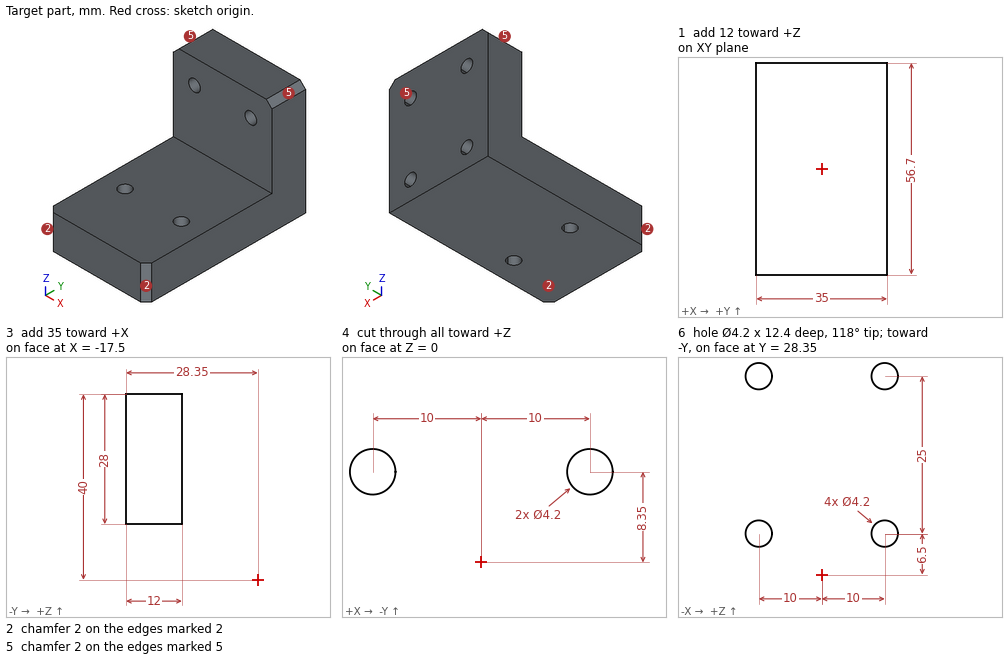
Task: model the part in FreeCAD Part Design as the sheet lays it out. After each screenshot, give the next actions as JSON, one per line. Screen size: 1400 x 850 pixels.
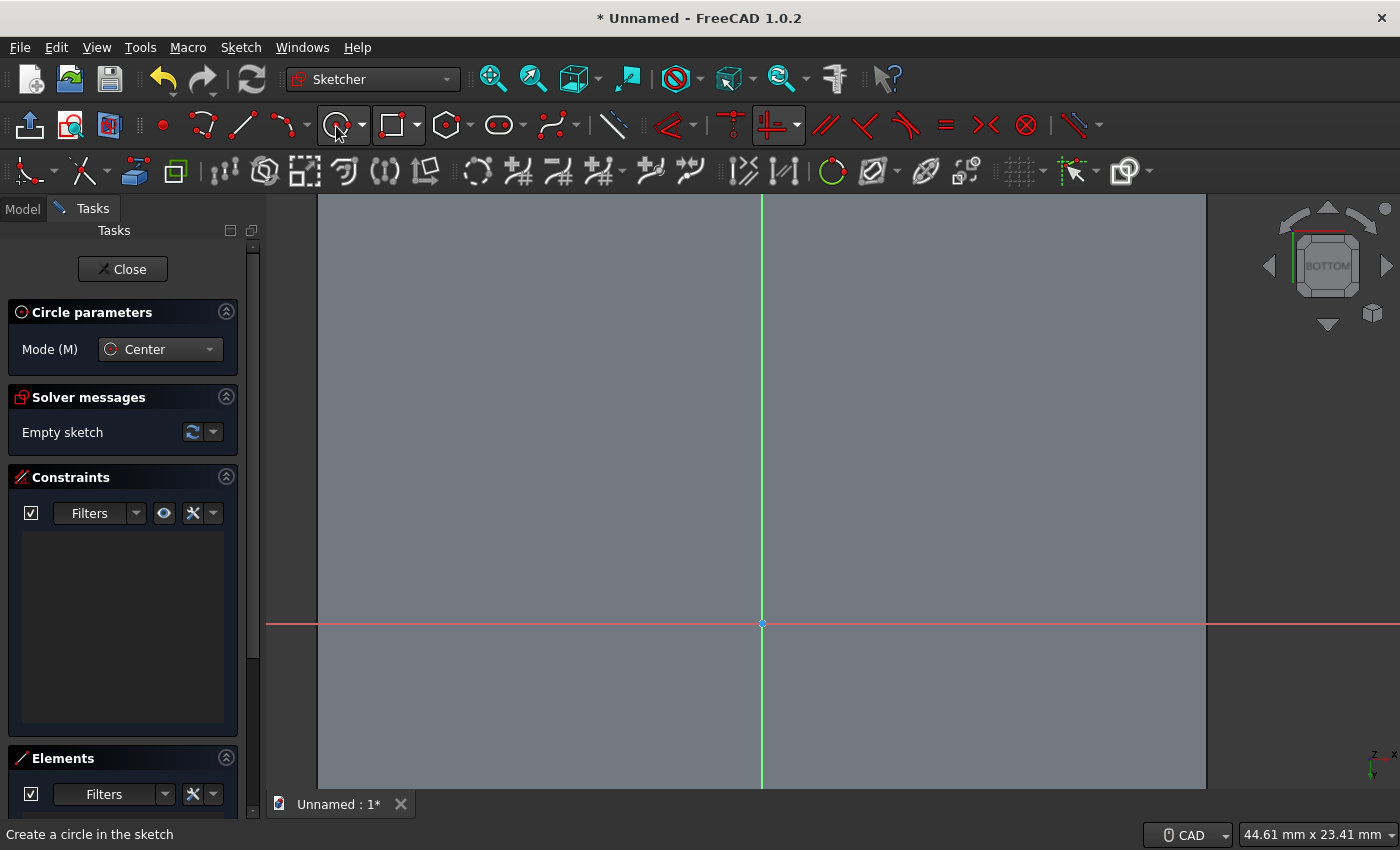
{"action": "left_click", "coordinate": [1016, 412]}
{"action": "left_click", "coordinate": [1054, 374]}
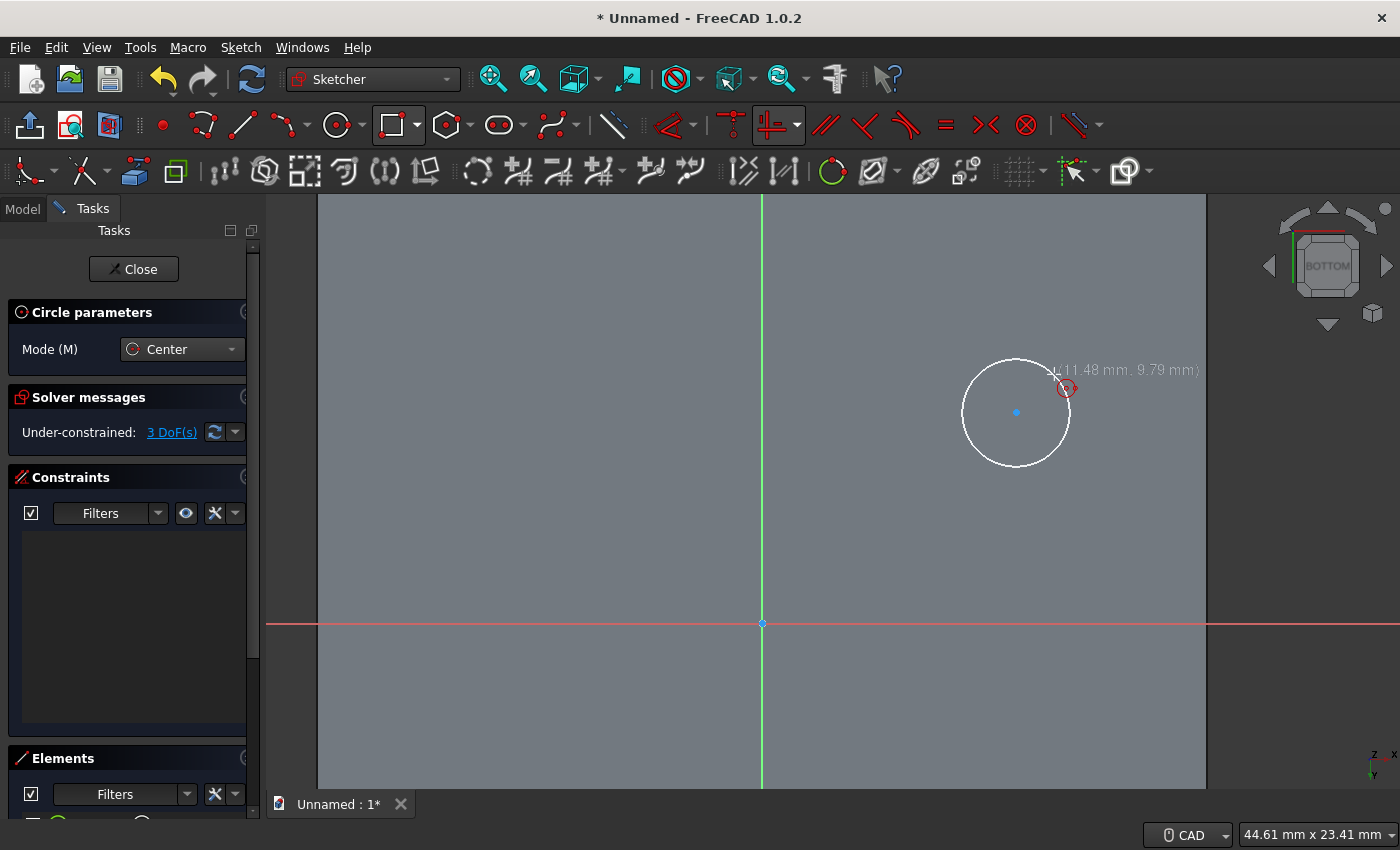
{"action": "left_click", "coordinate": [508, 412]}
{"action": "left_click", "coordinate": [546, 374]}
{"action": "key", "text": "Escape"}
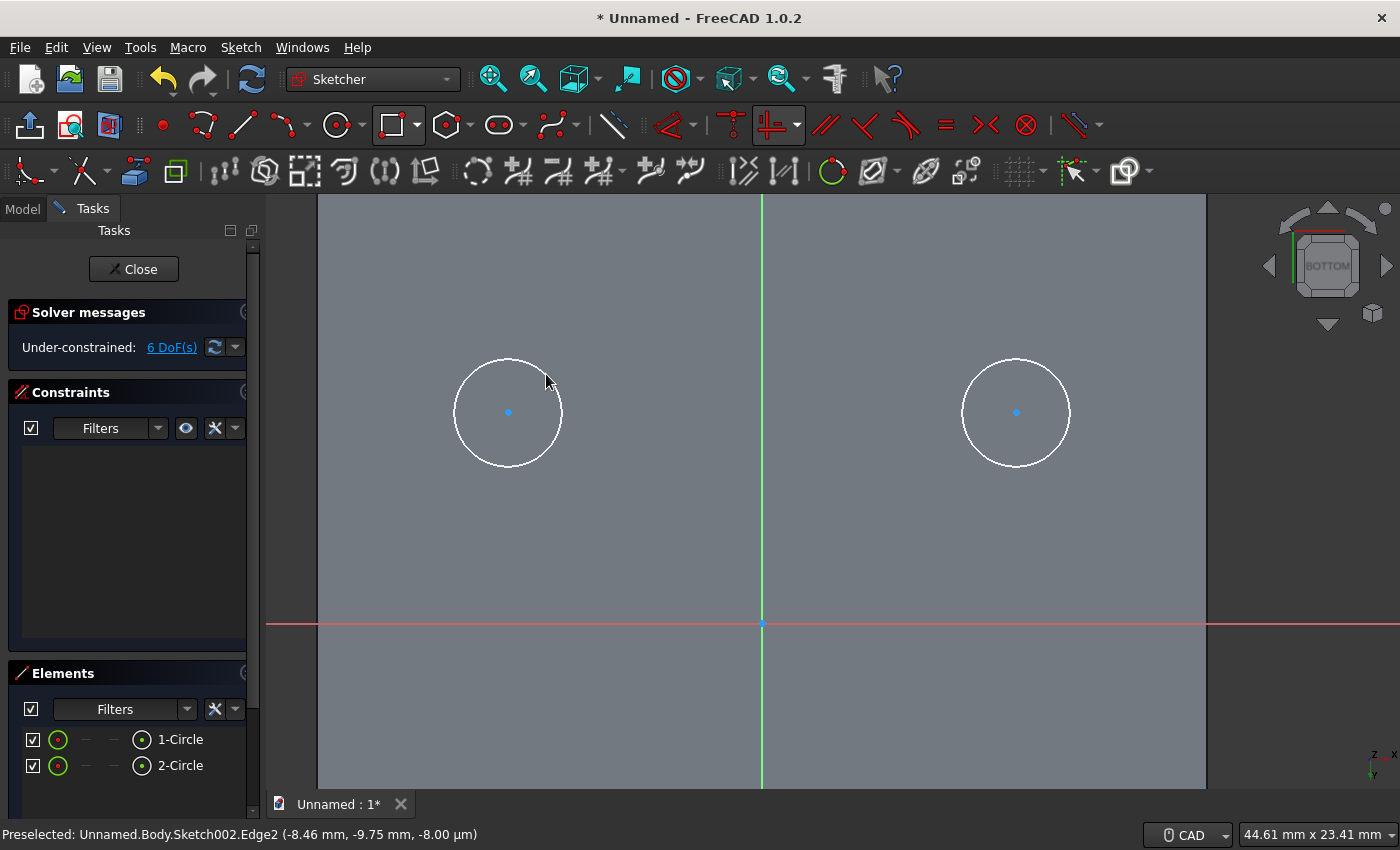
{"action": "left_click", "coordinate": [1054, 375]}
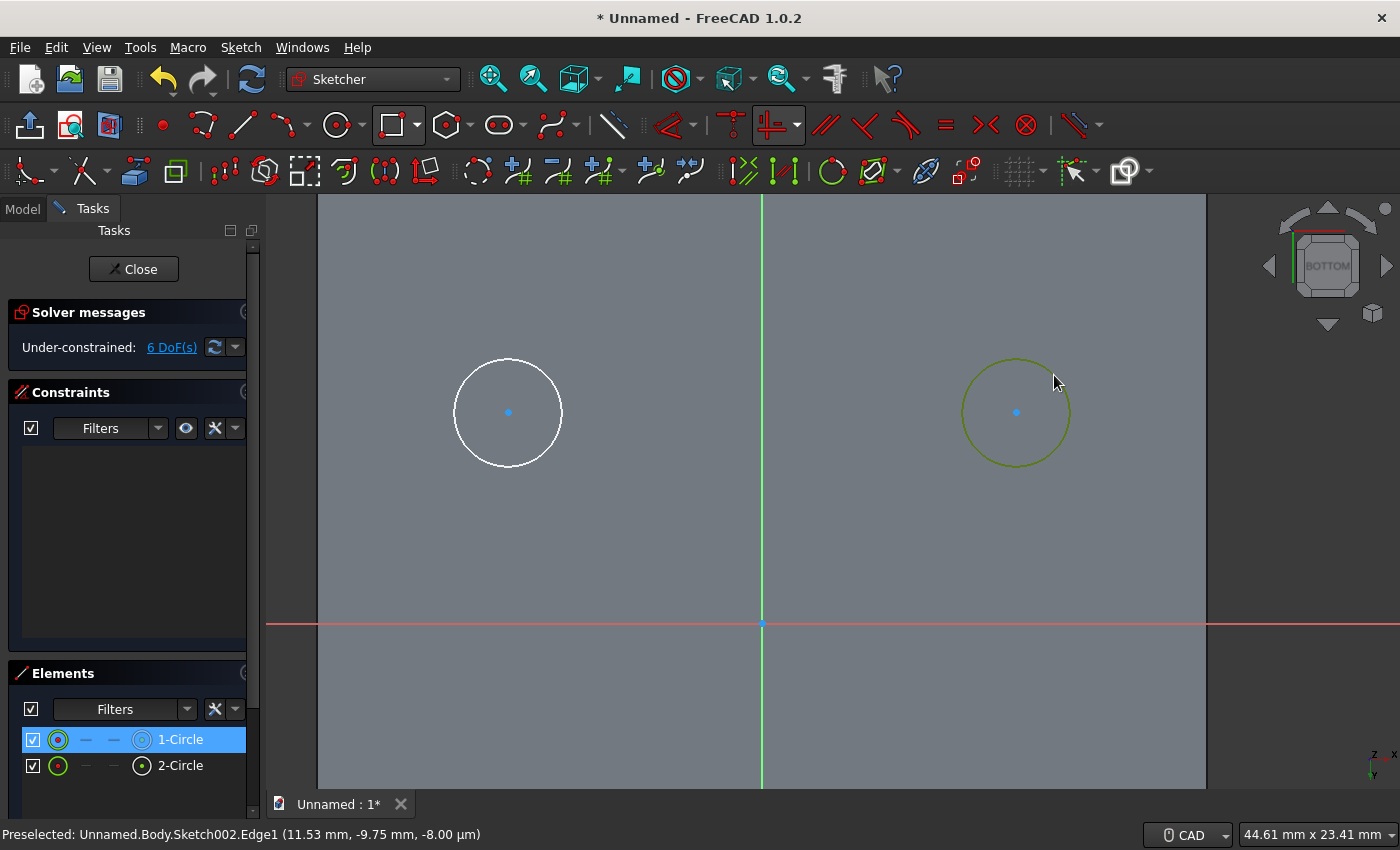
{"action": "left_click", "coordinate": [546, 375]}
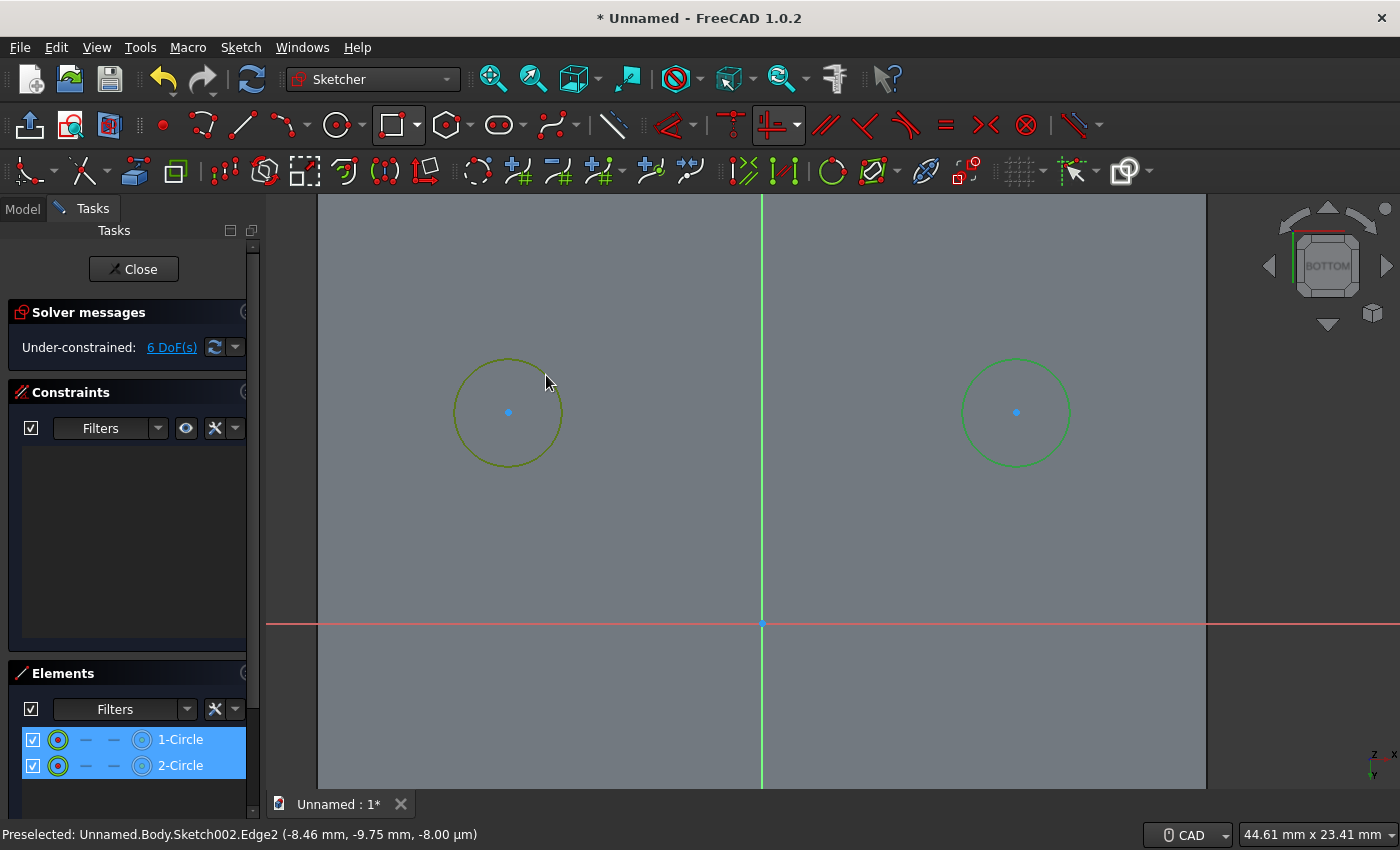
{"action": "left_click", "coordinate": [946, 126]}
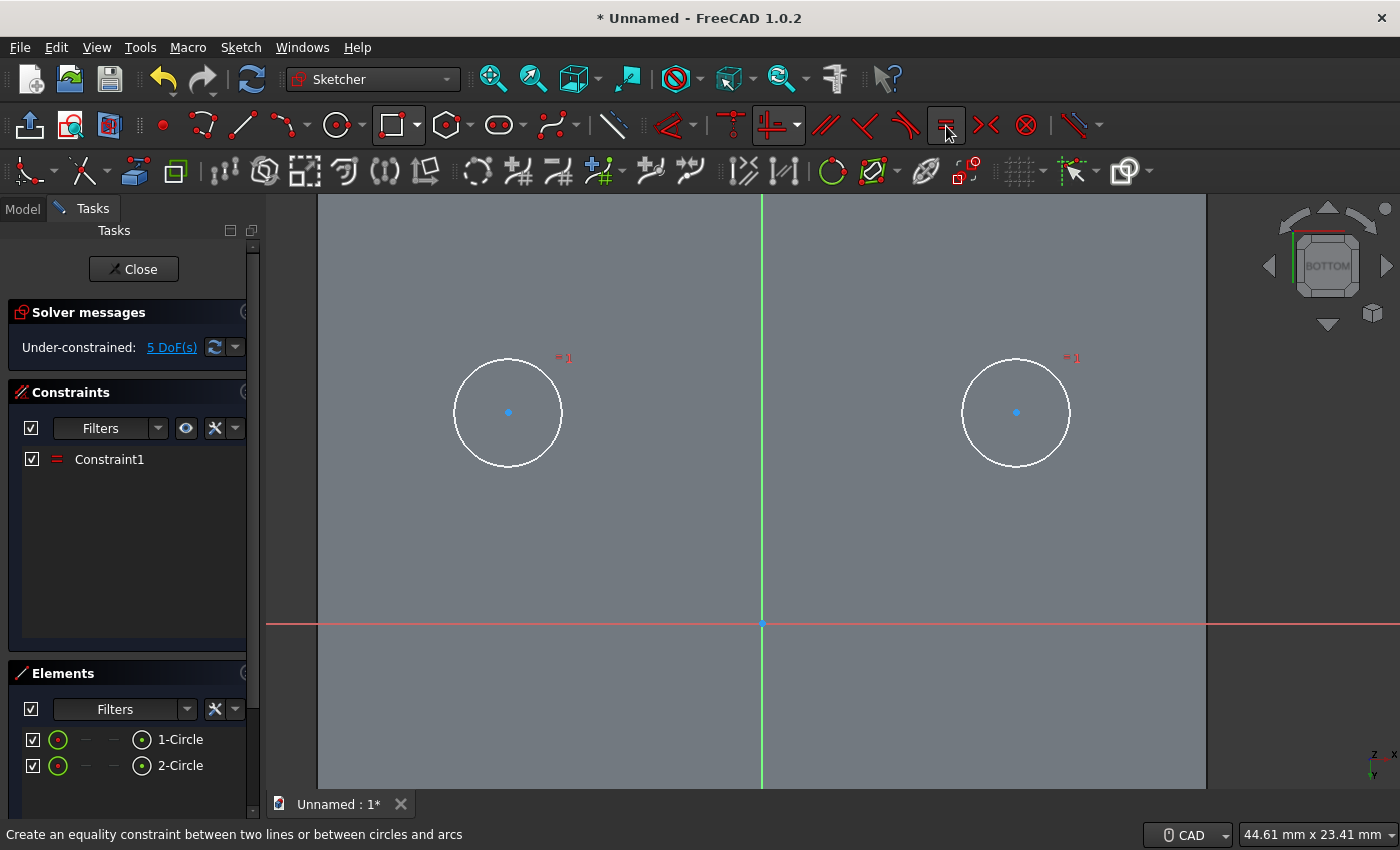
{"action": "left_click", "coordinate": [1016, 413]}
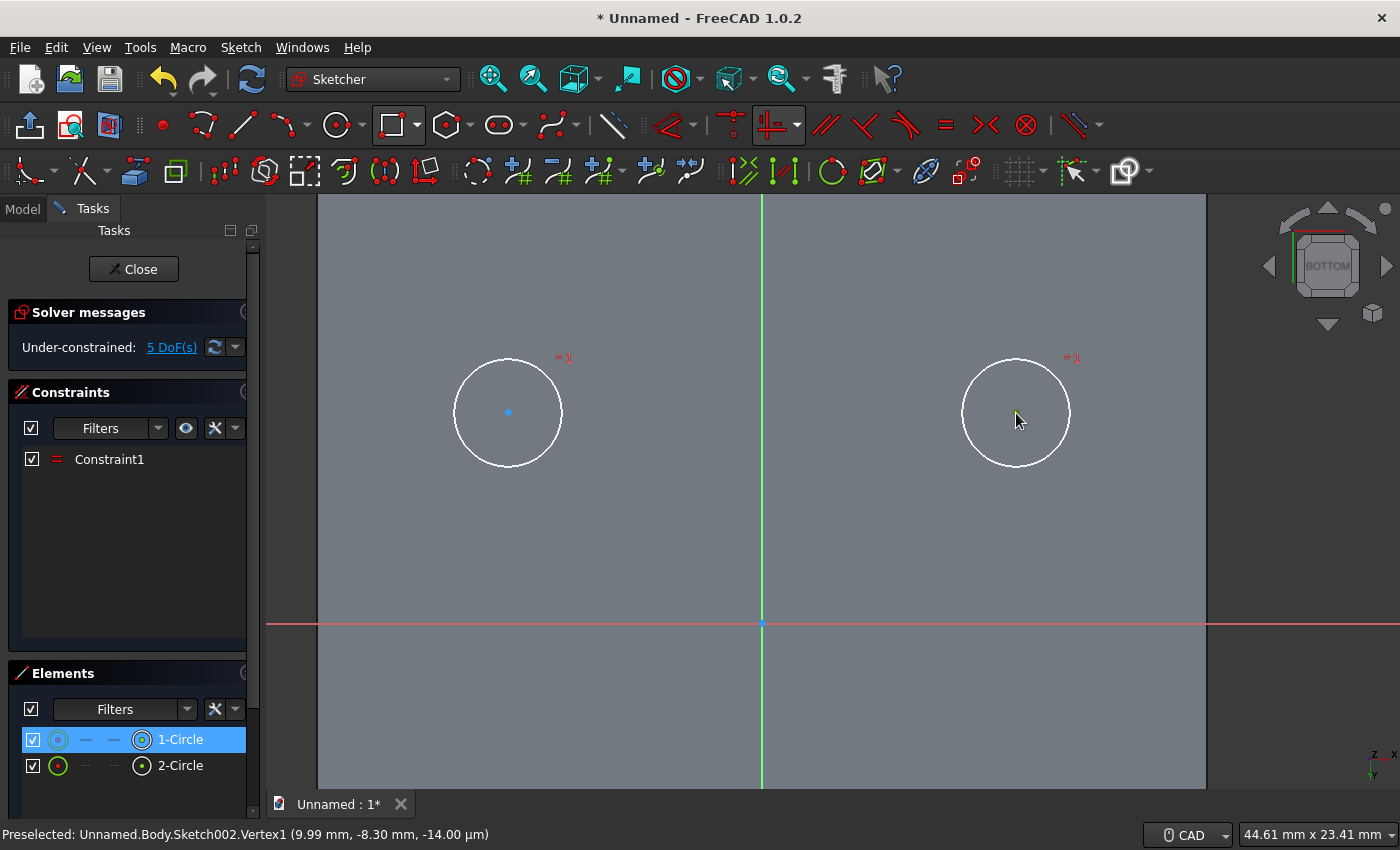
{"action": "left_click", "coordinate": [508, 413]}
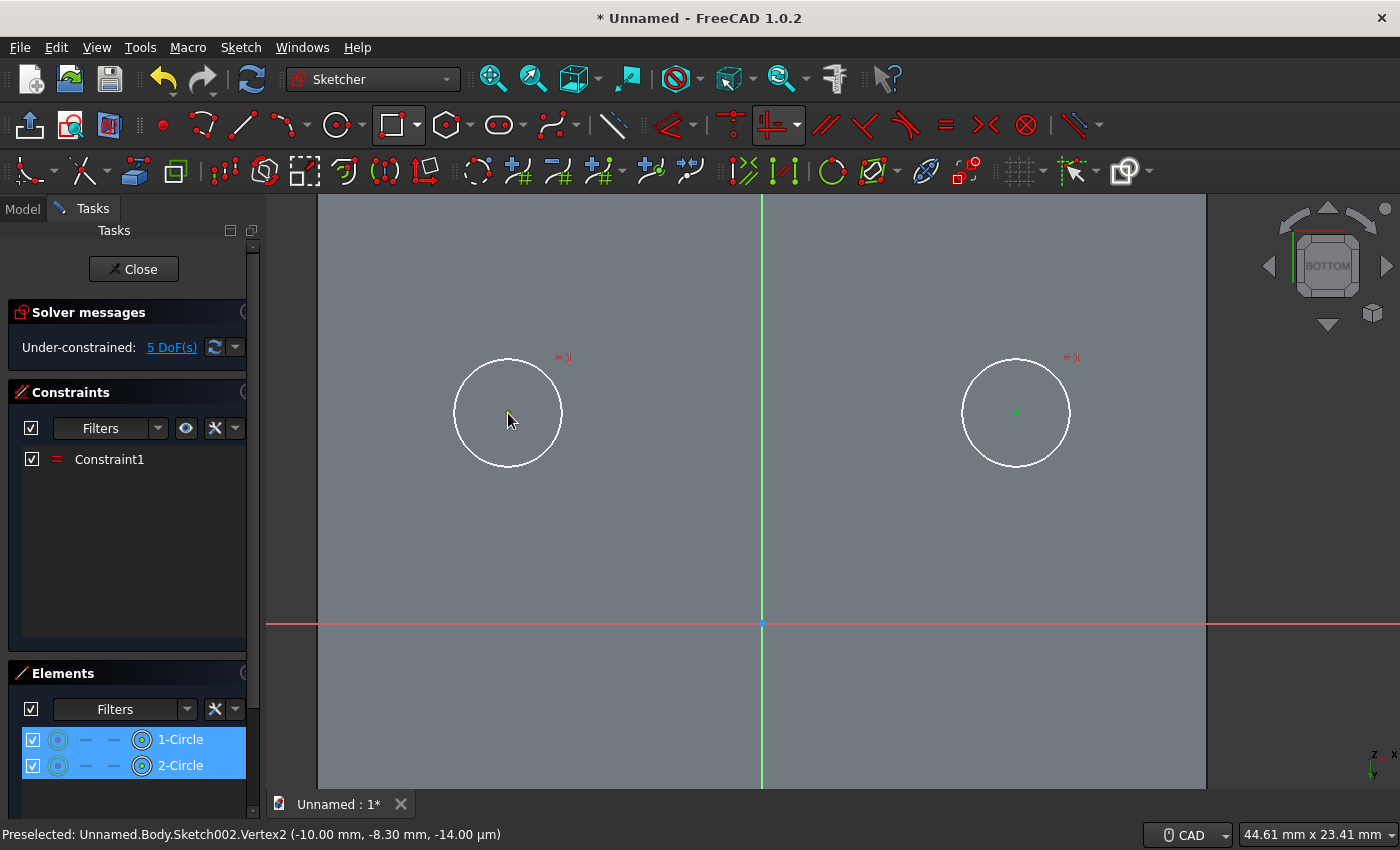
{"action": "left_click", "coordinate": [800, 126]}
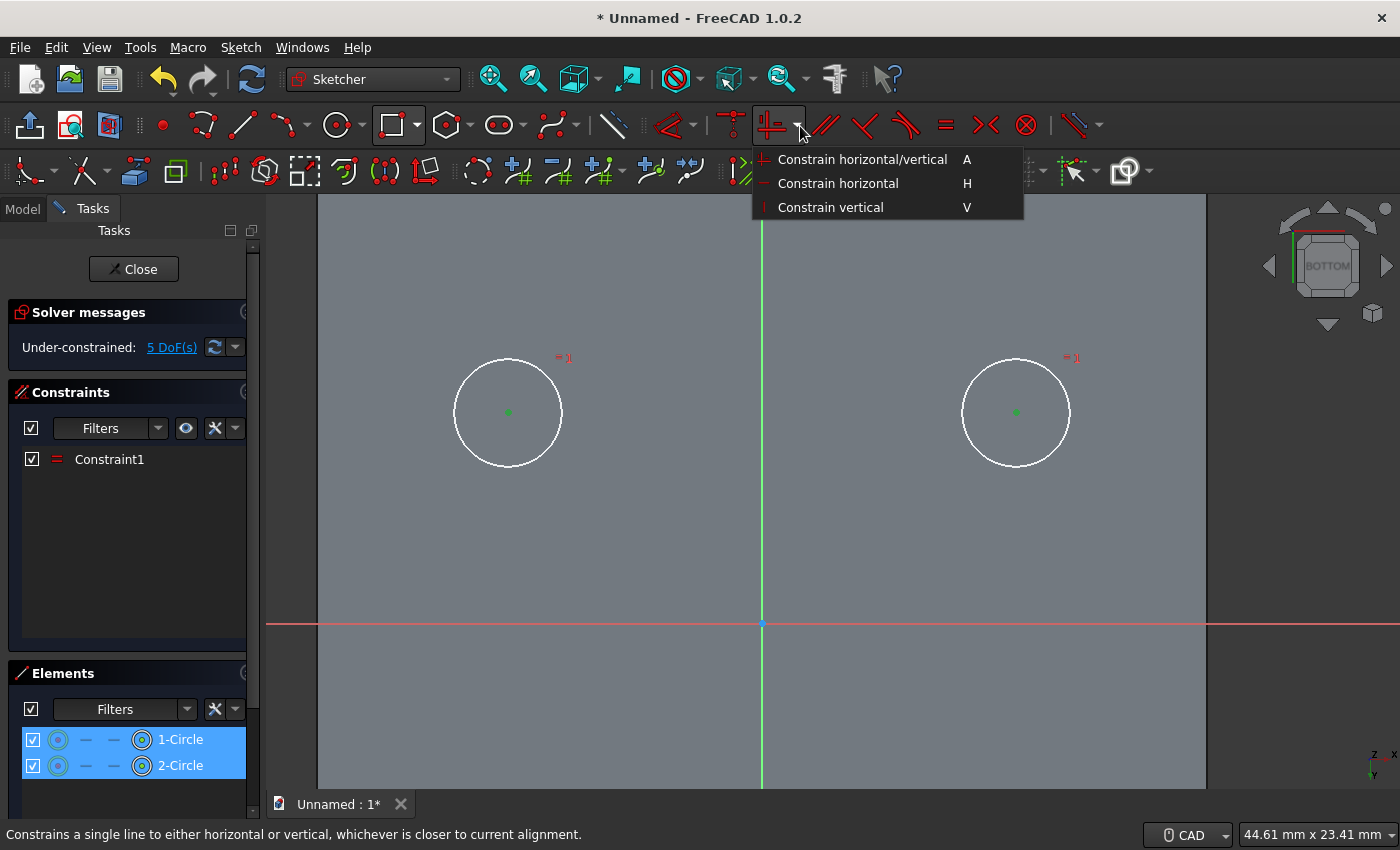
{"action": "left_click", "coordinate": [888, 183]}